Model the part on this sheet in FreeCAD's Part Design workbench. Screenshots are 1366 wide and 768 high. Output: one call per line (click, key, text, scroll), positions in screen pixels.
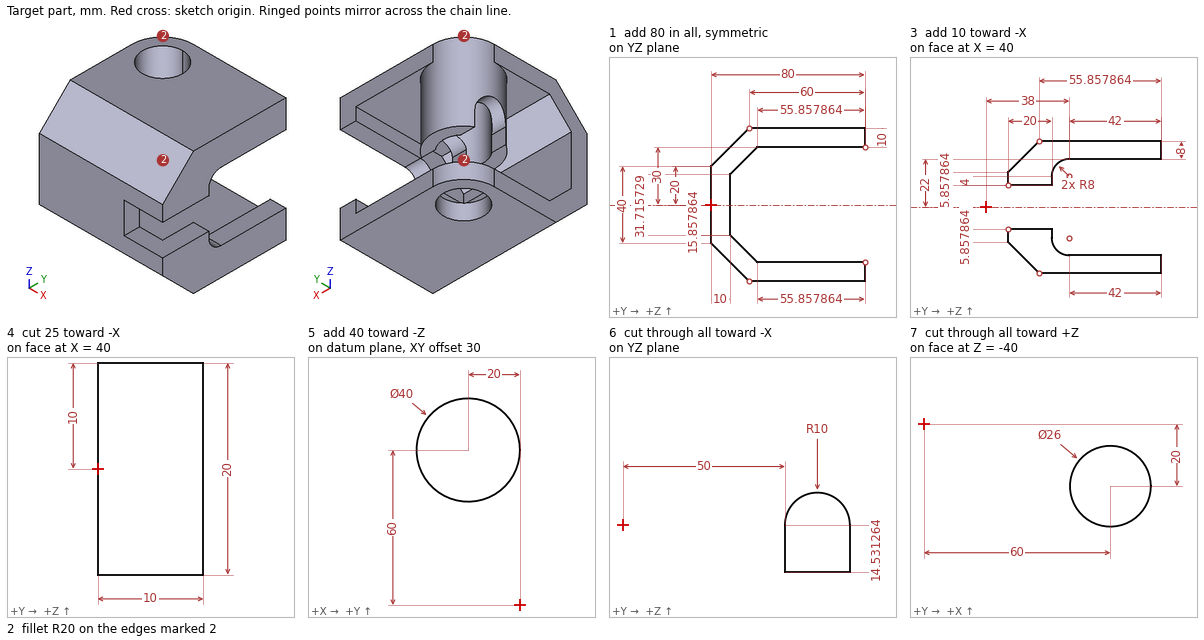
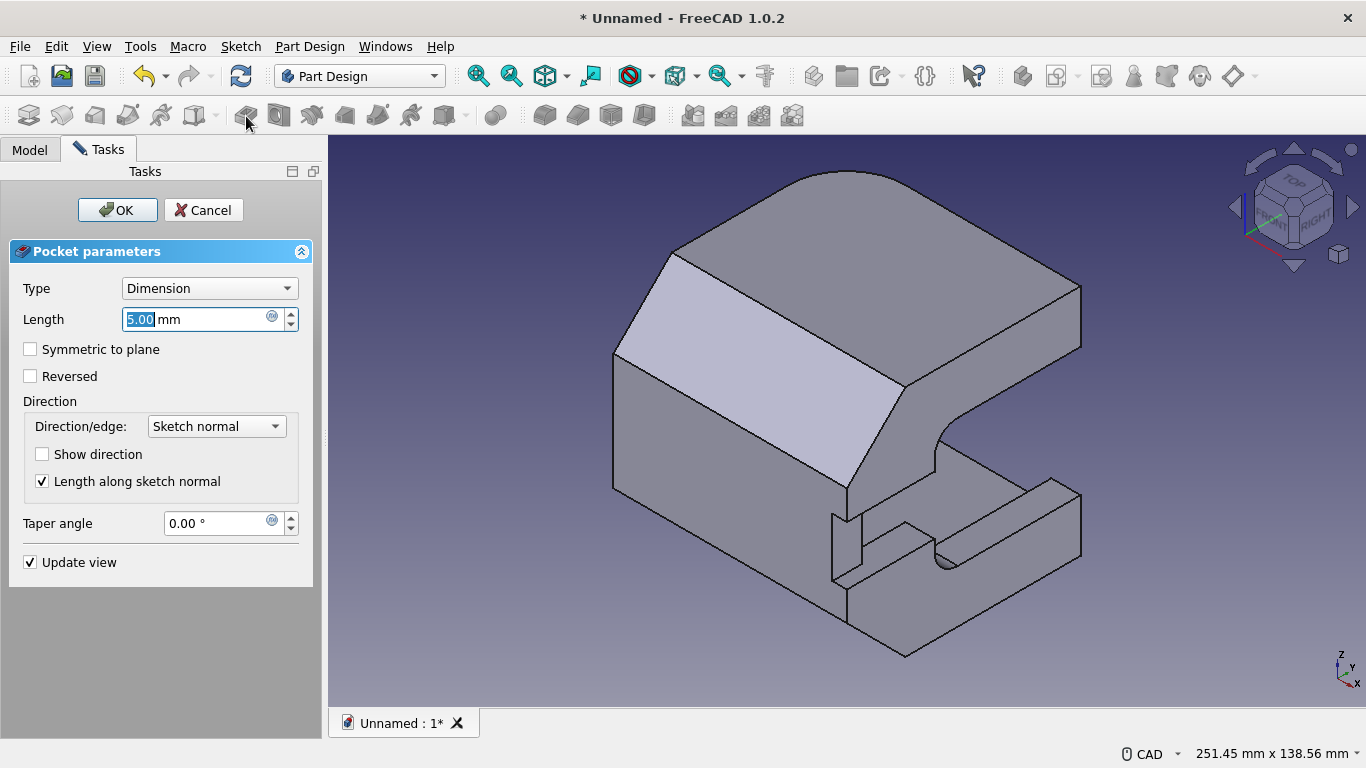
text(25)
key(Tab)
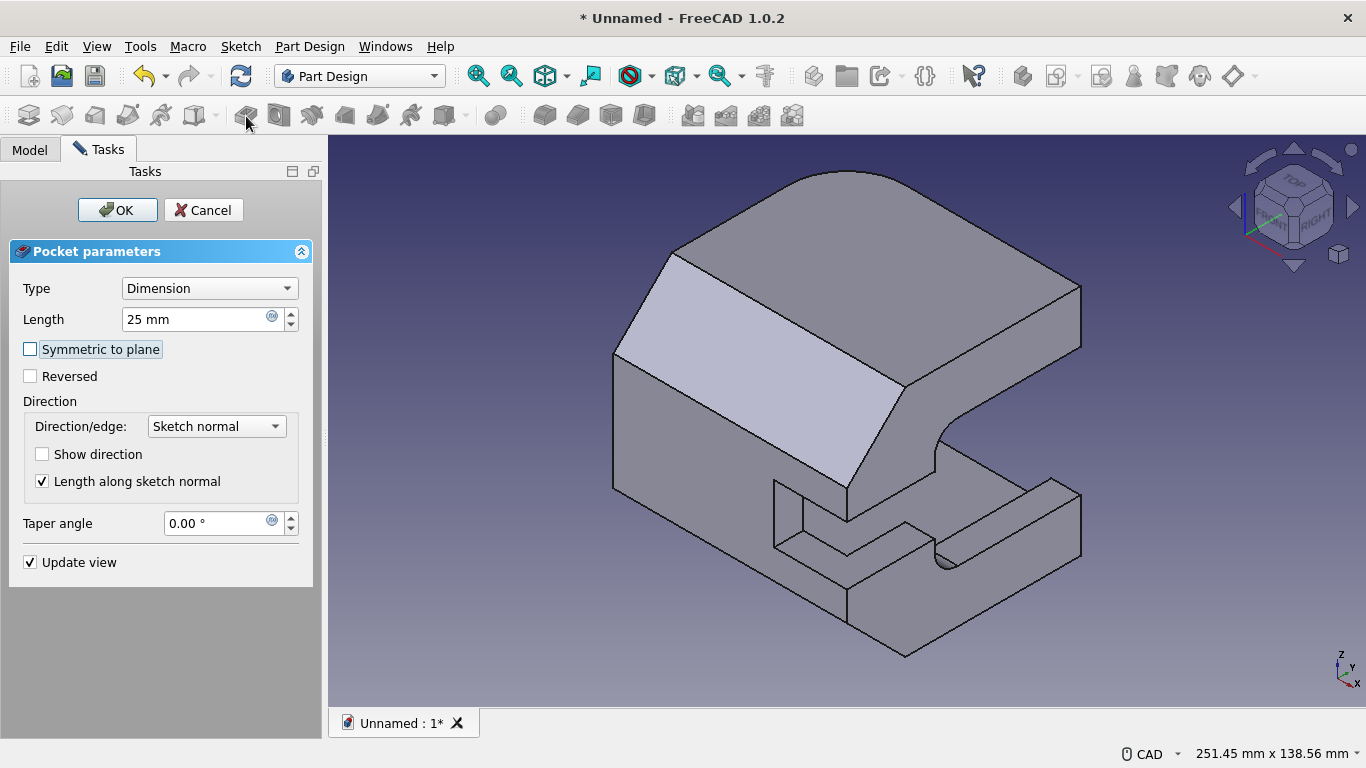
click(118, 210)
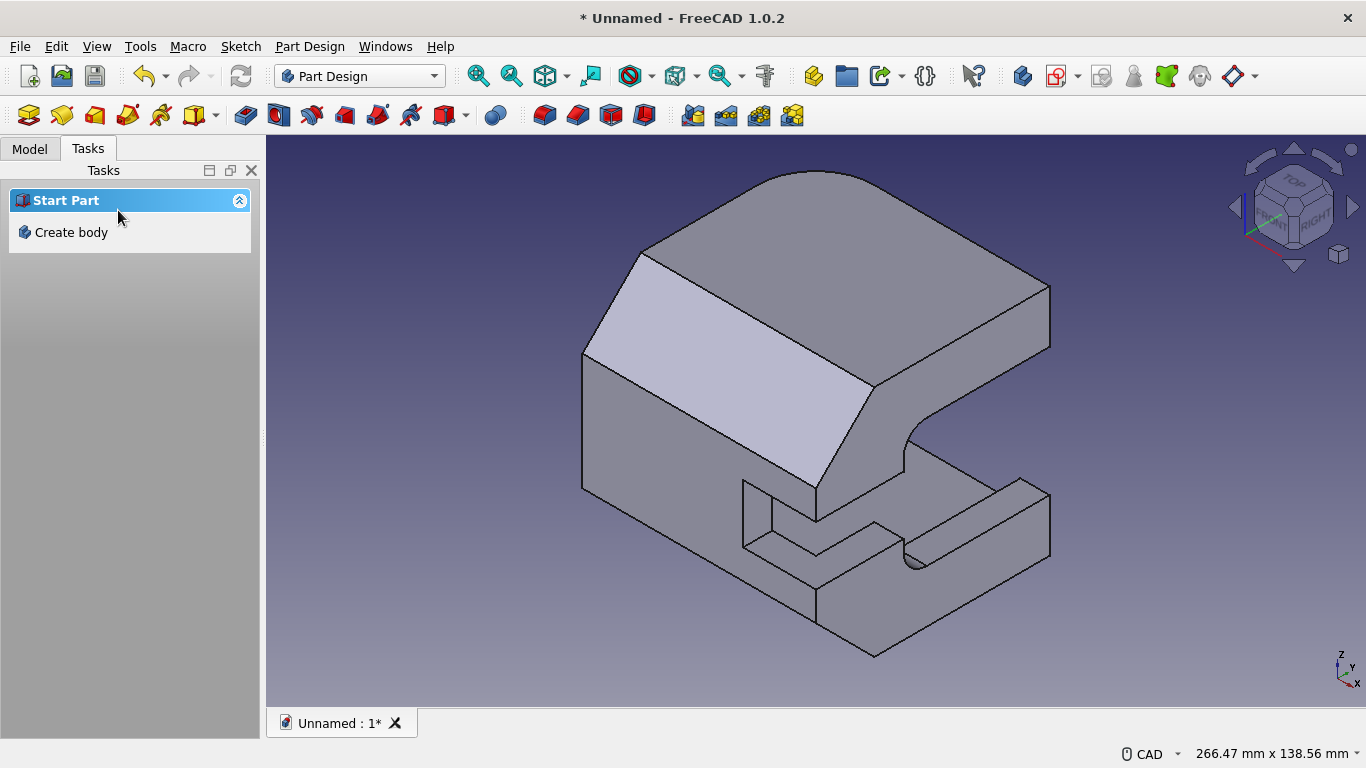
click(30, 148)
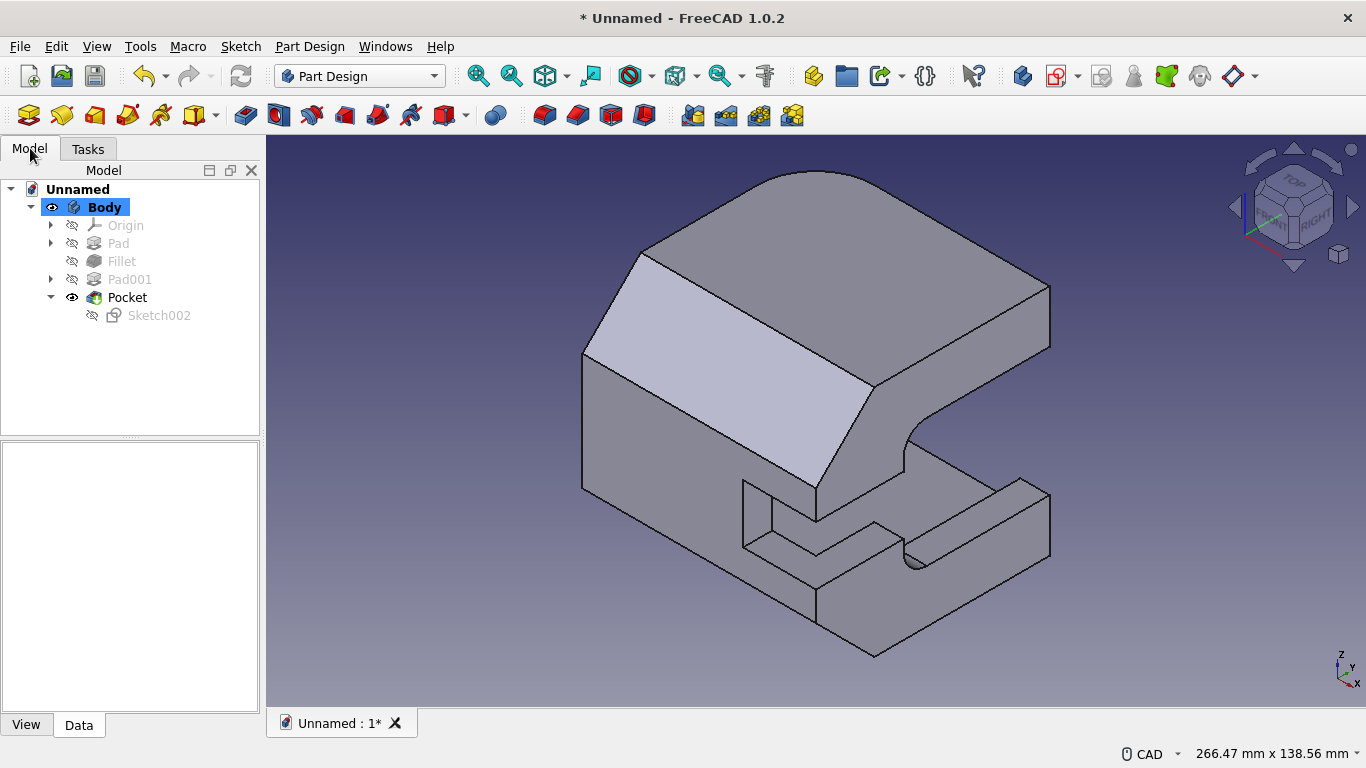
click(51, 225)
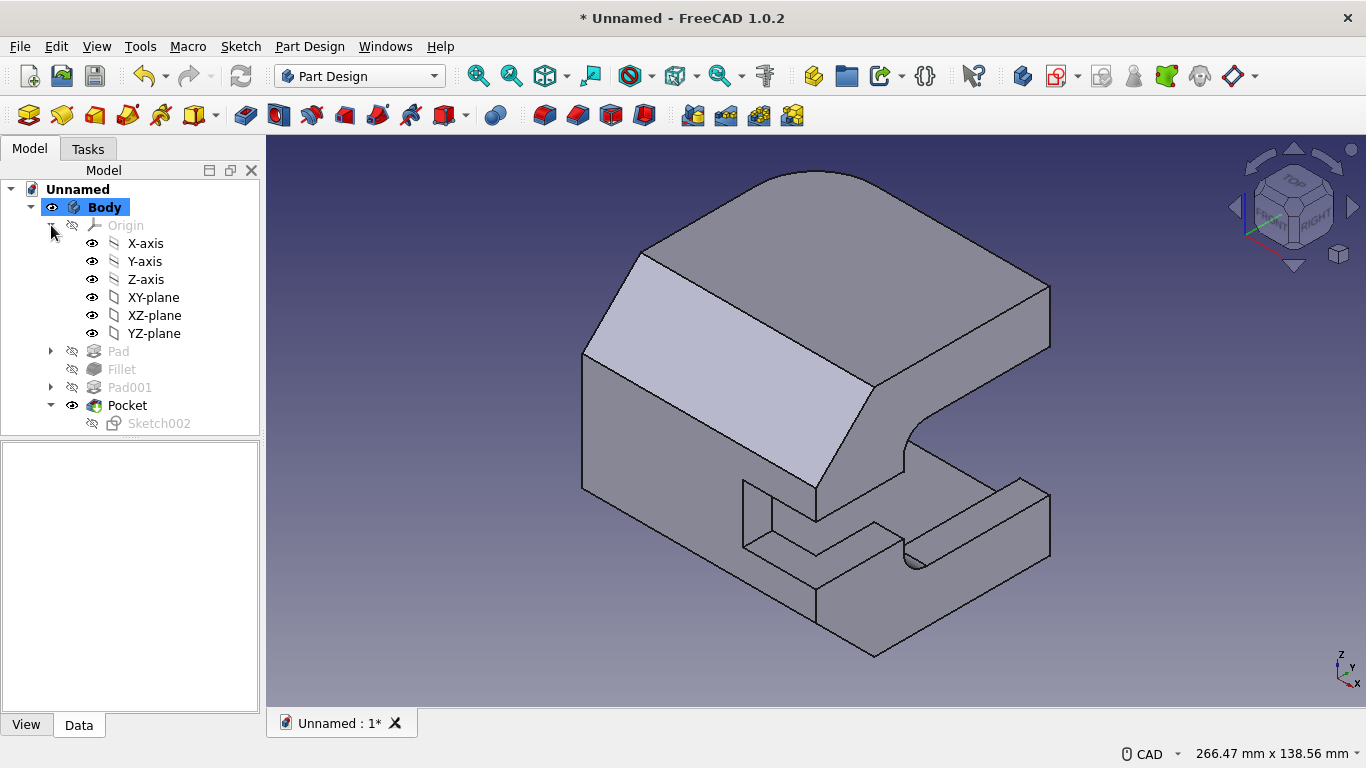
click(137, 297)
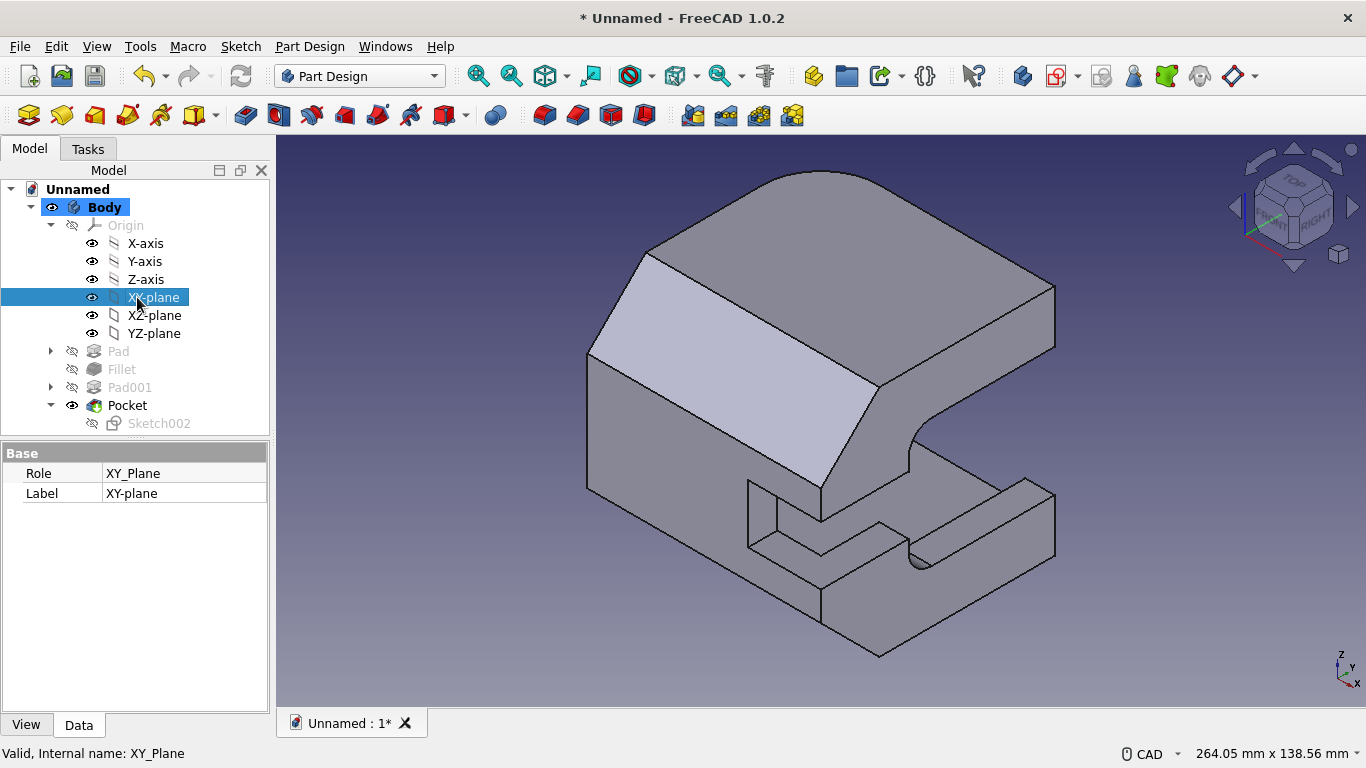
click(1232, 76)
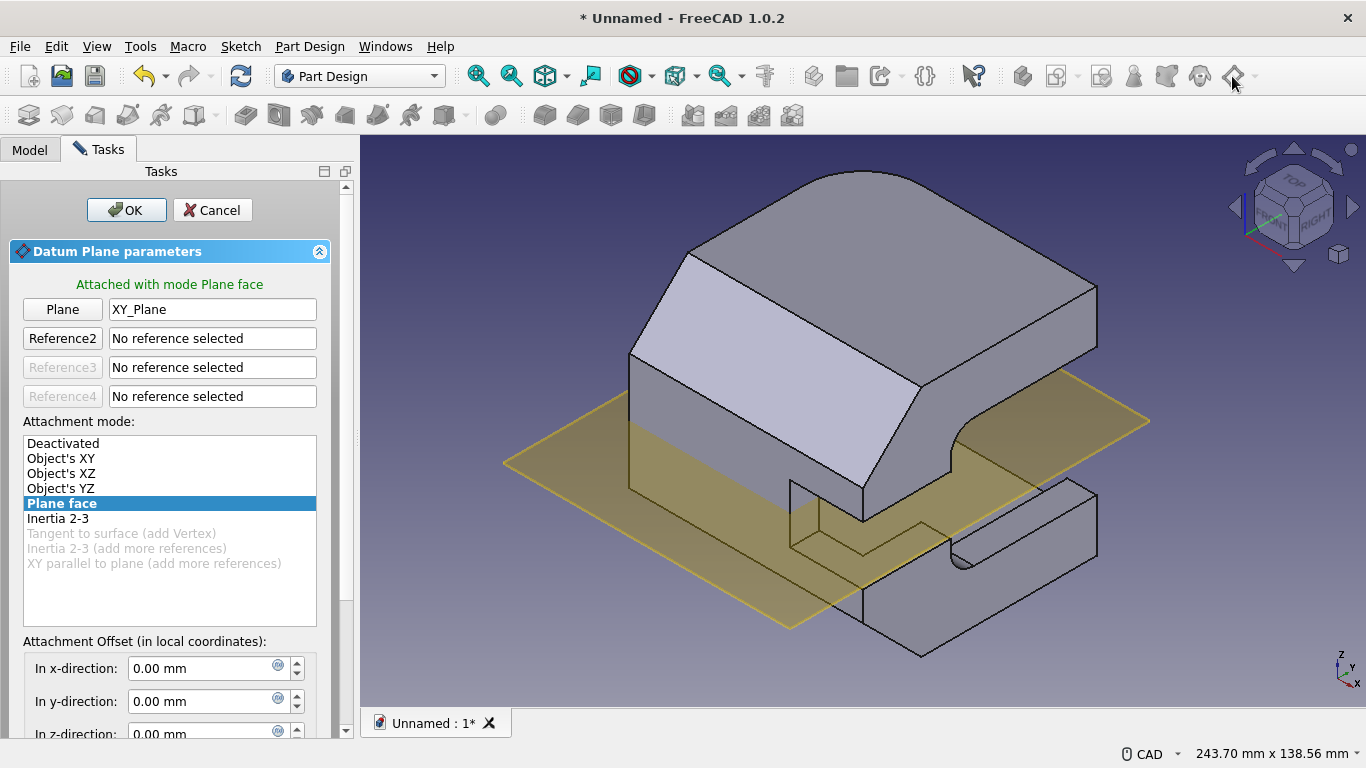
scroll(346, 460, down, 2)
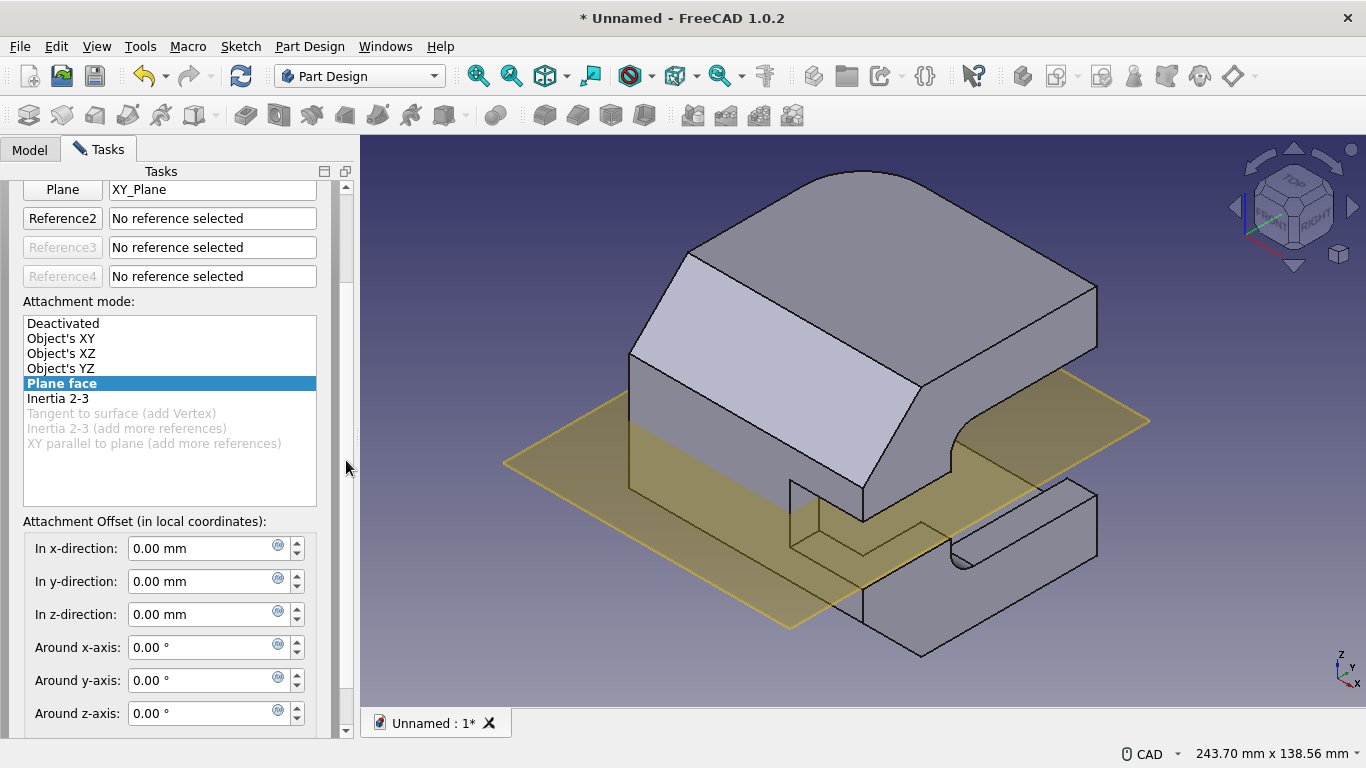
triple_click(210, 614)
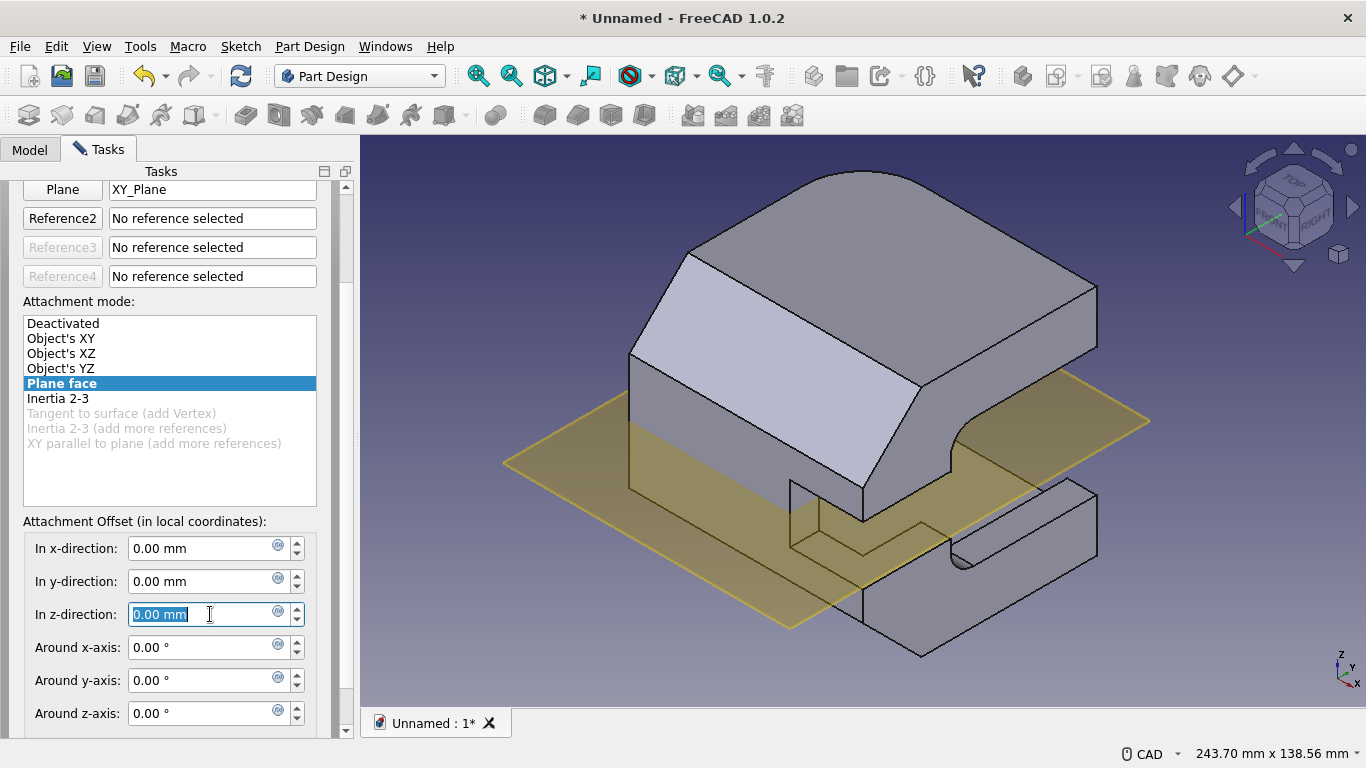
text(30)
key(Tab)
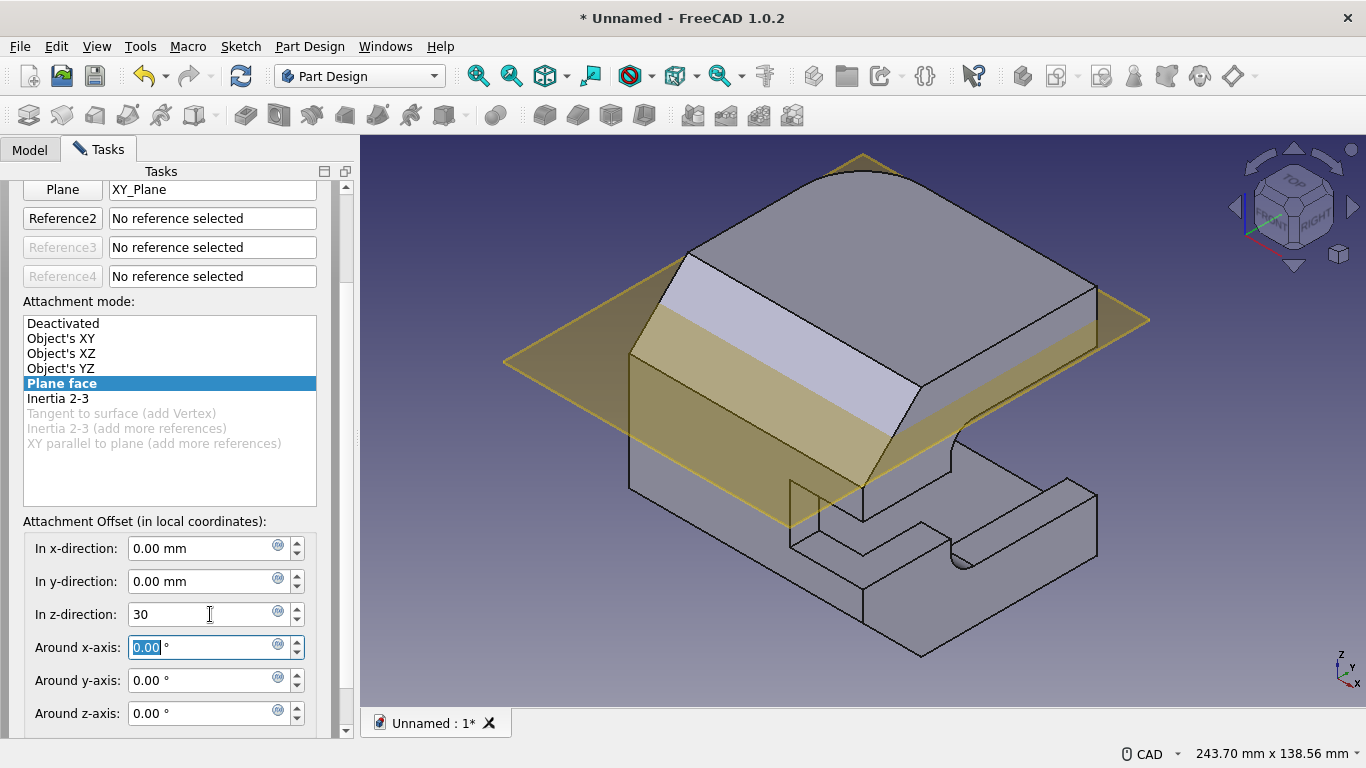
scroll(346, 460, up, 3)